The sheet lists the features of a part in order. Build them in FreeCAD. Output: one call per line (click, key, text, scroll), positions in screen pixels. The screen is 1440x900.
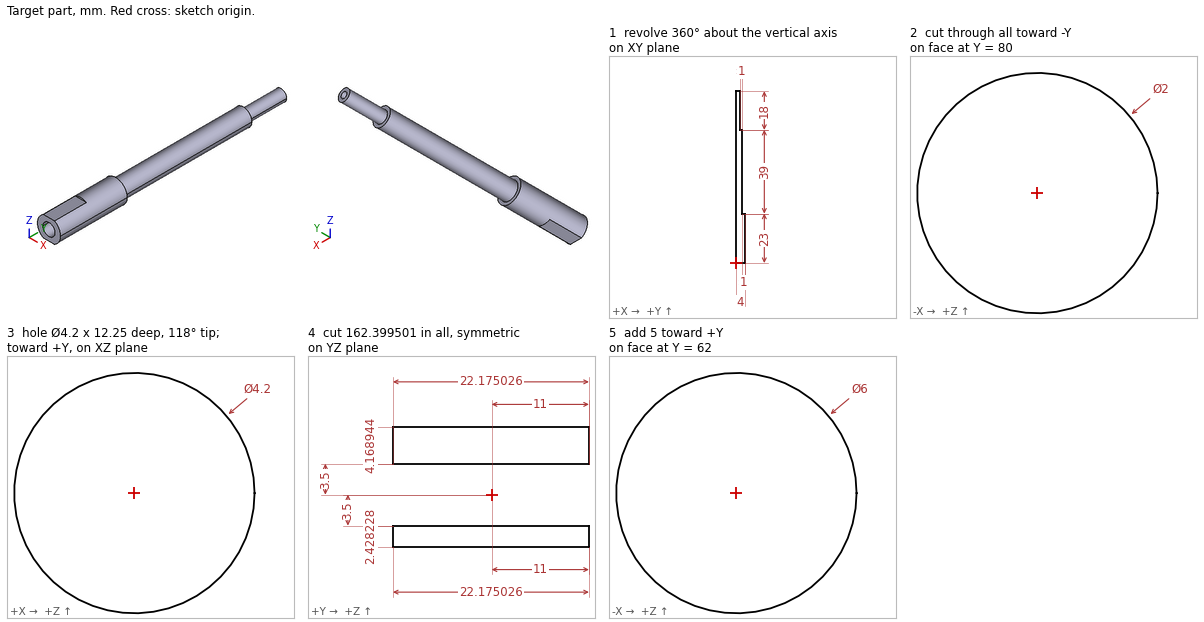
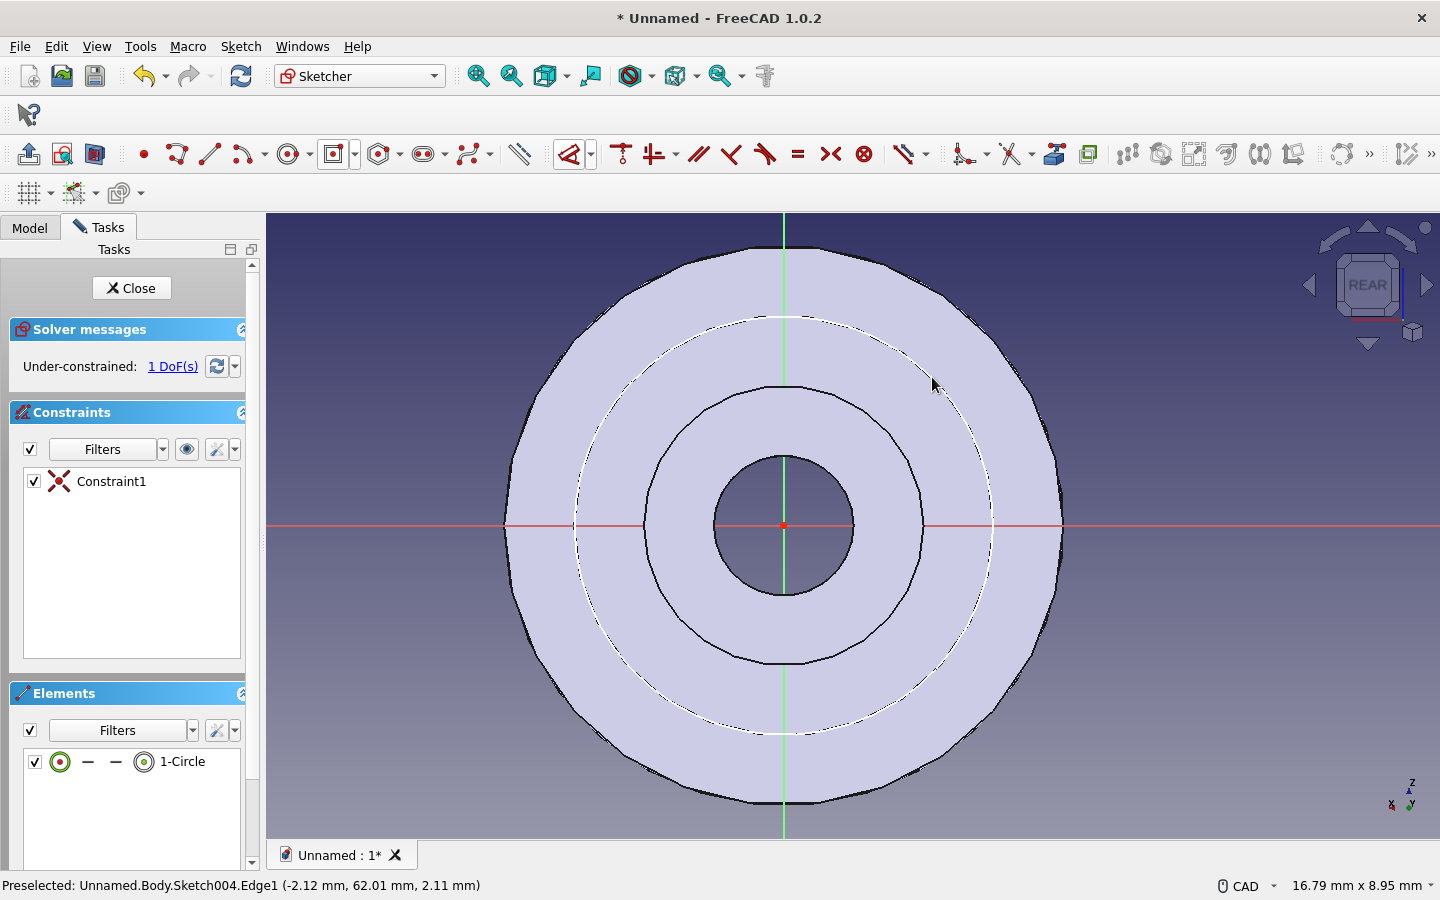
click(931, 377)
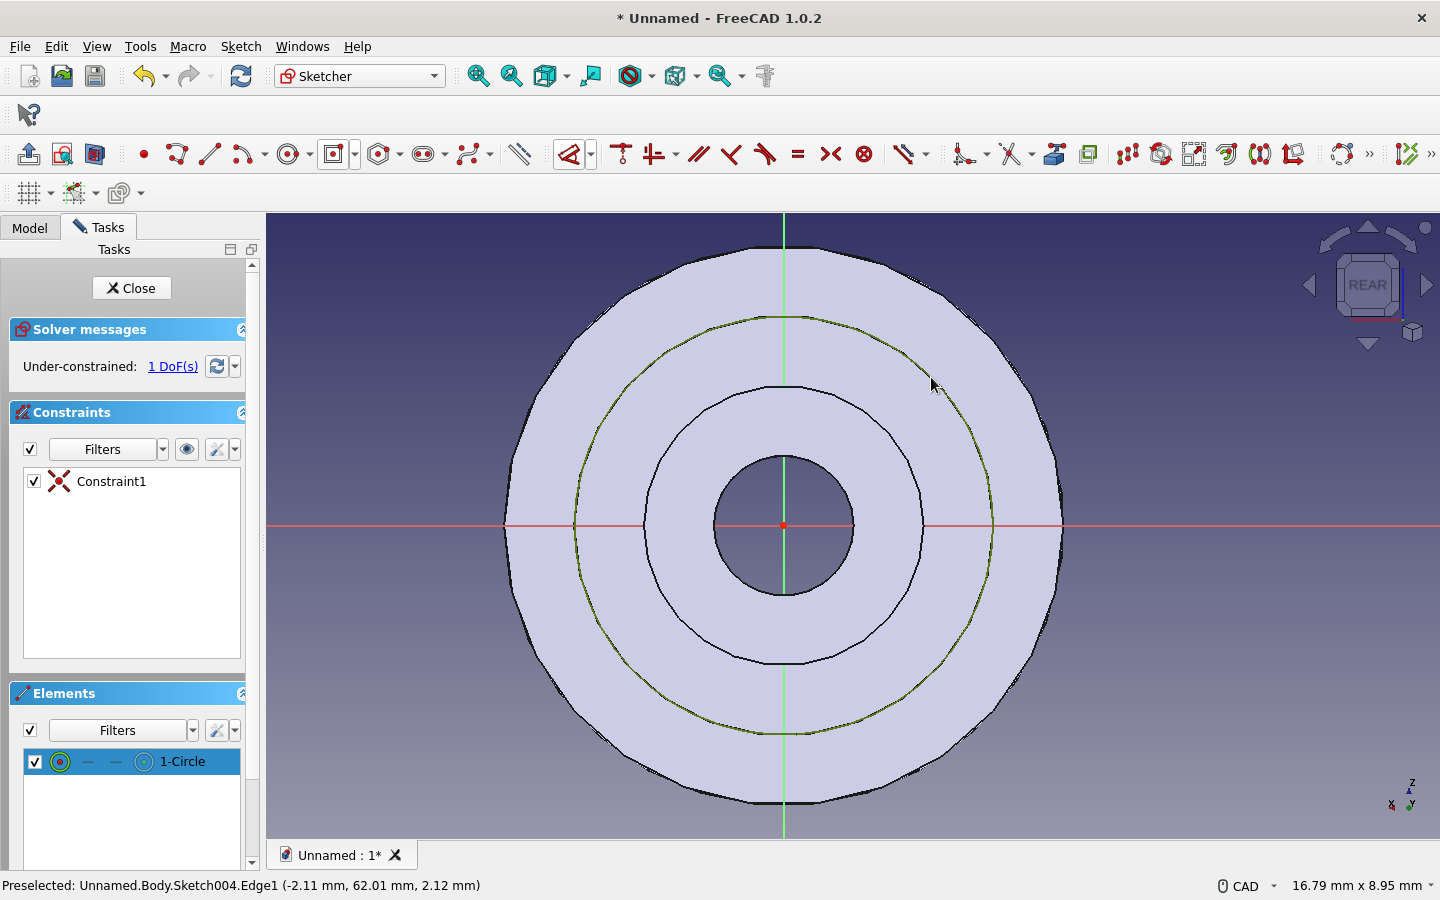
key(k)
key(o)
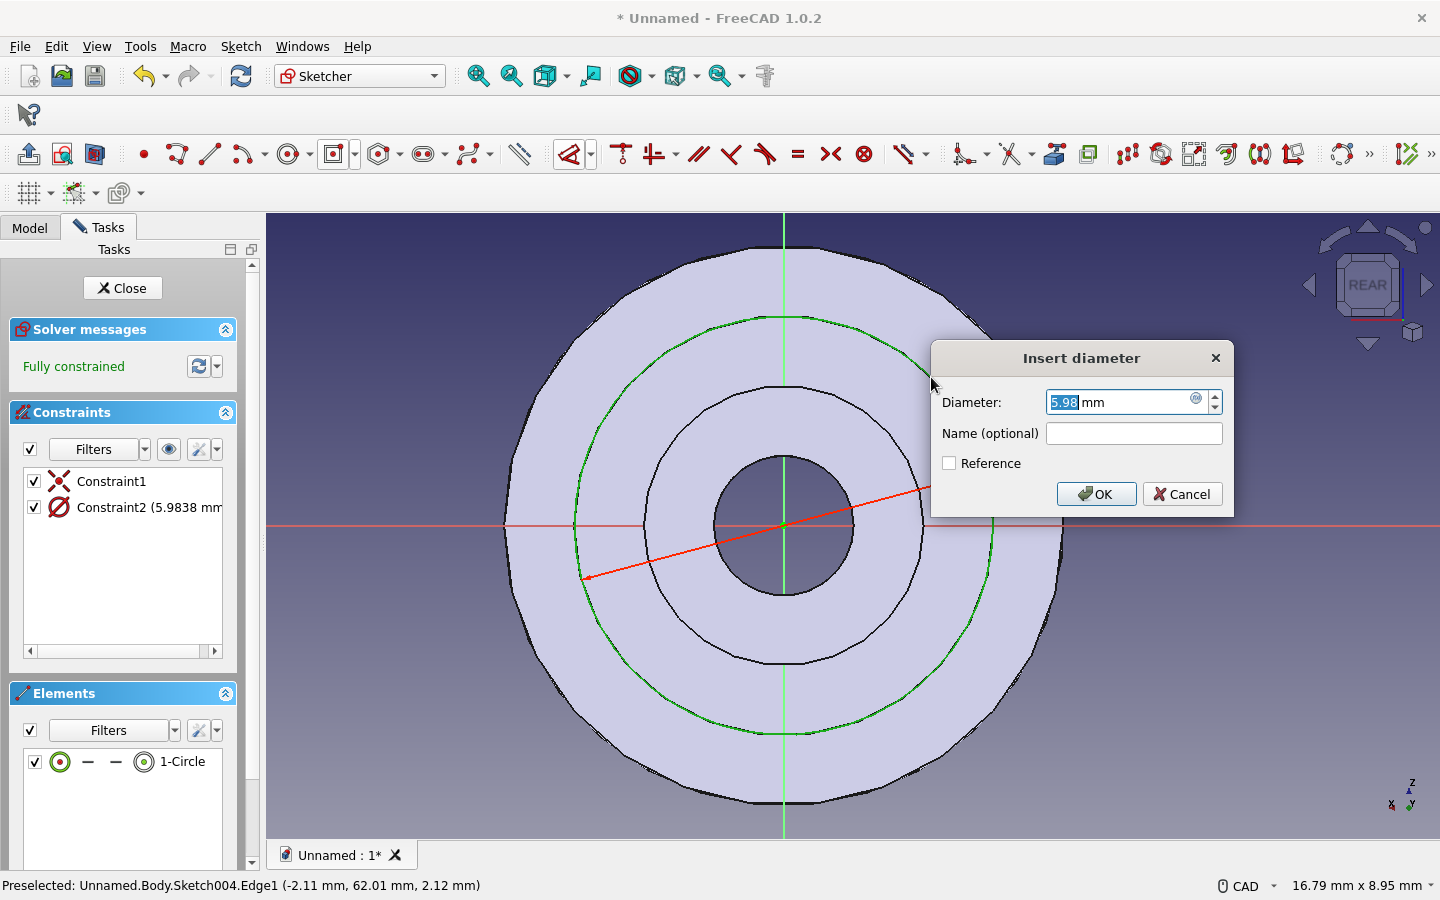
text(6)
key(Return)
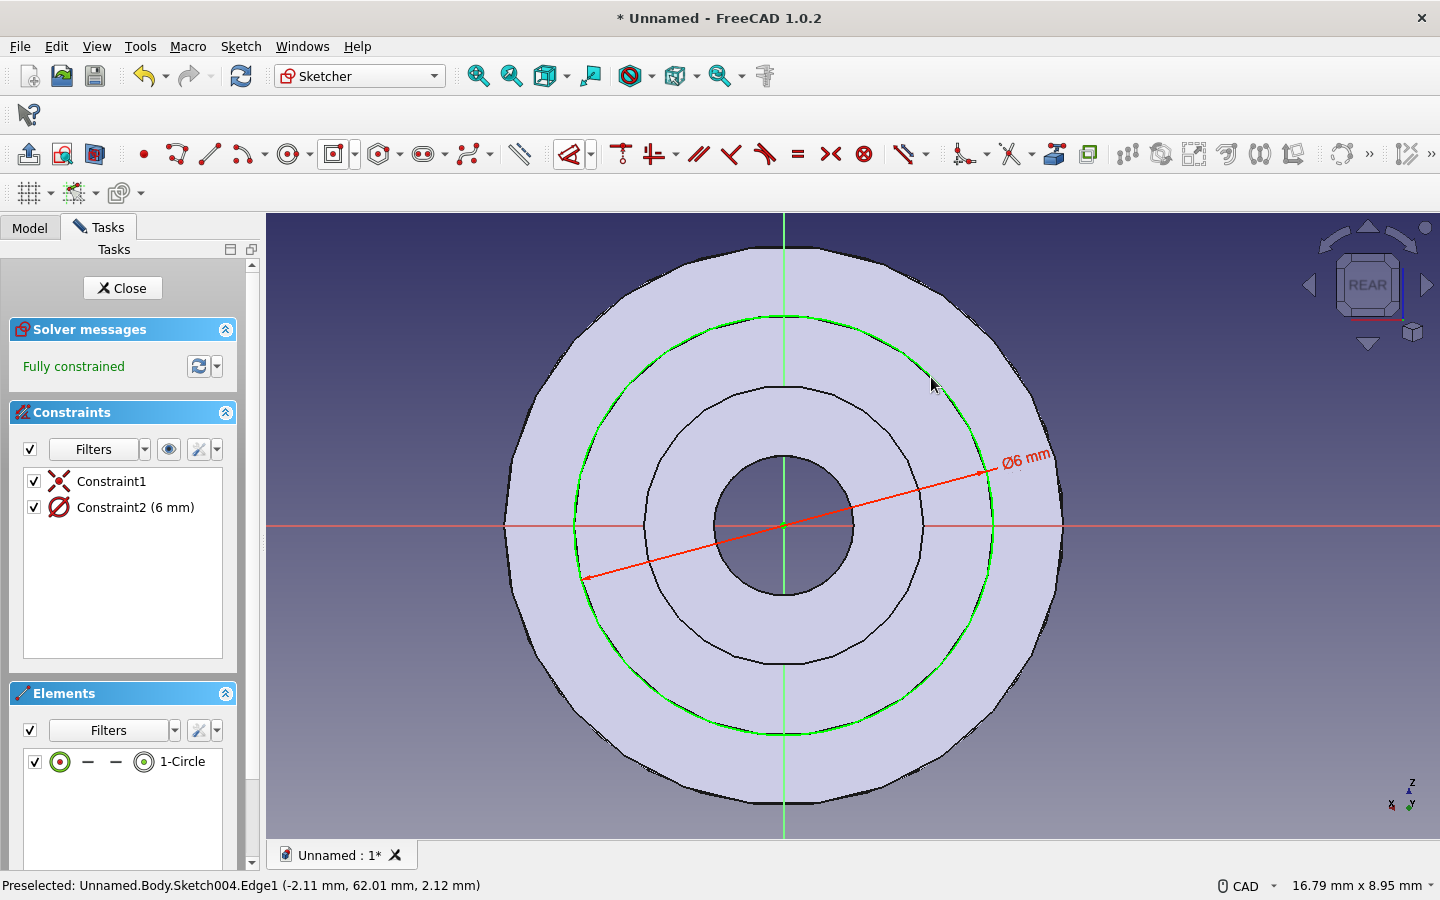
click(123, 288)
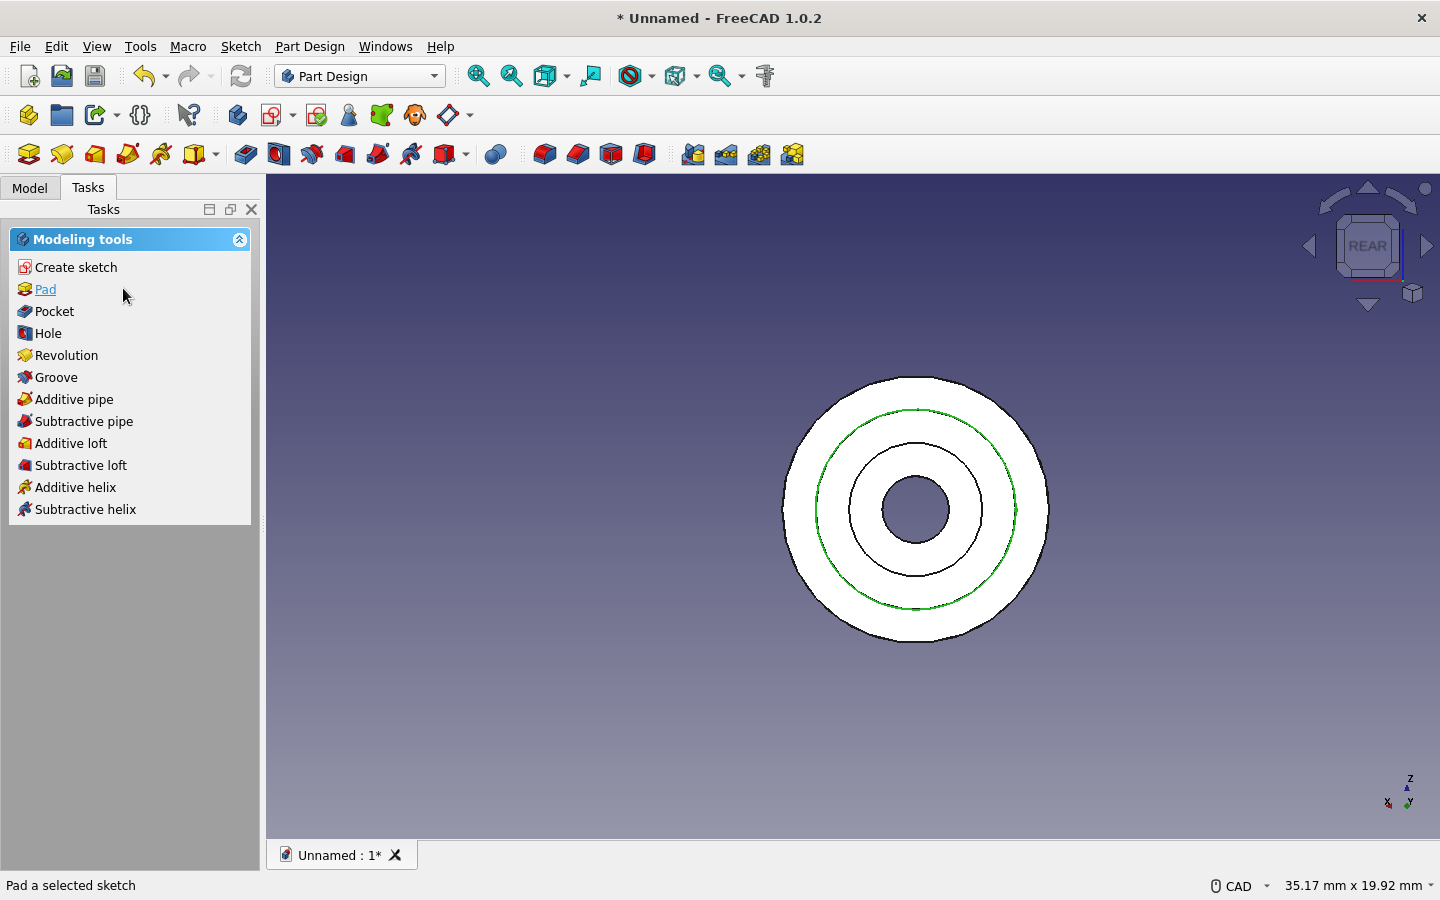
click(29, 154)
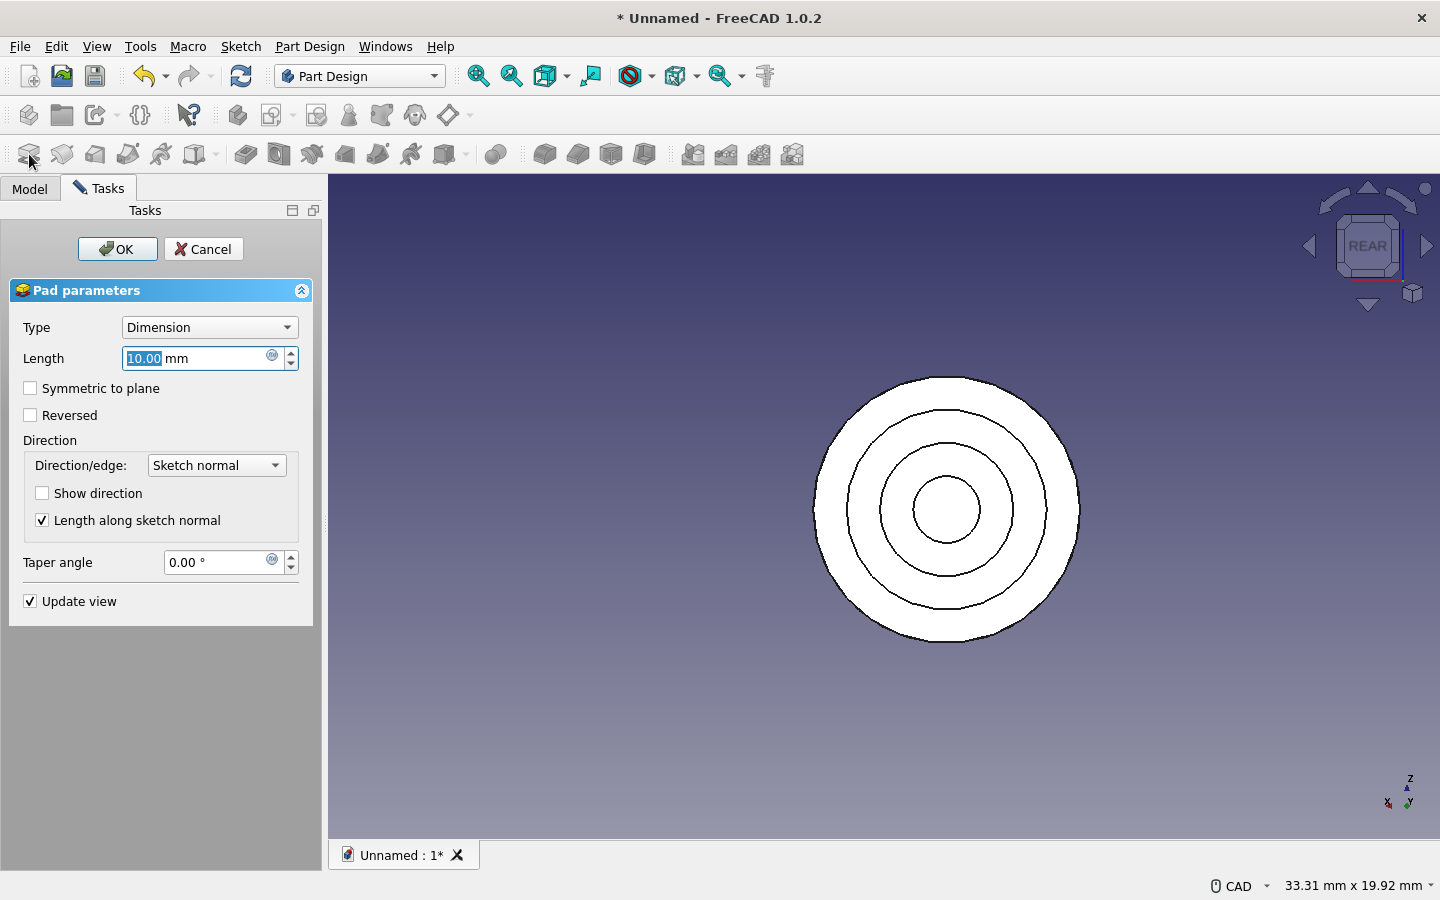
text(5)
key(Tab)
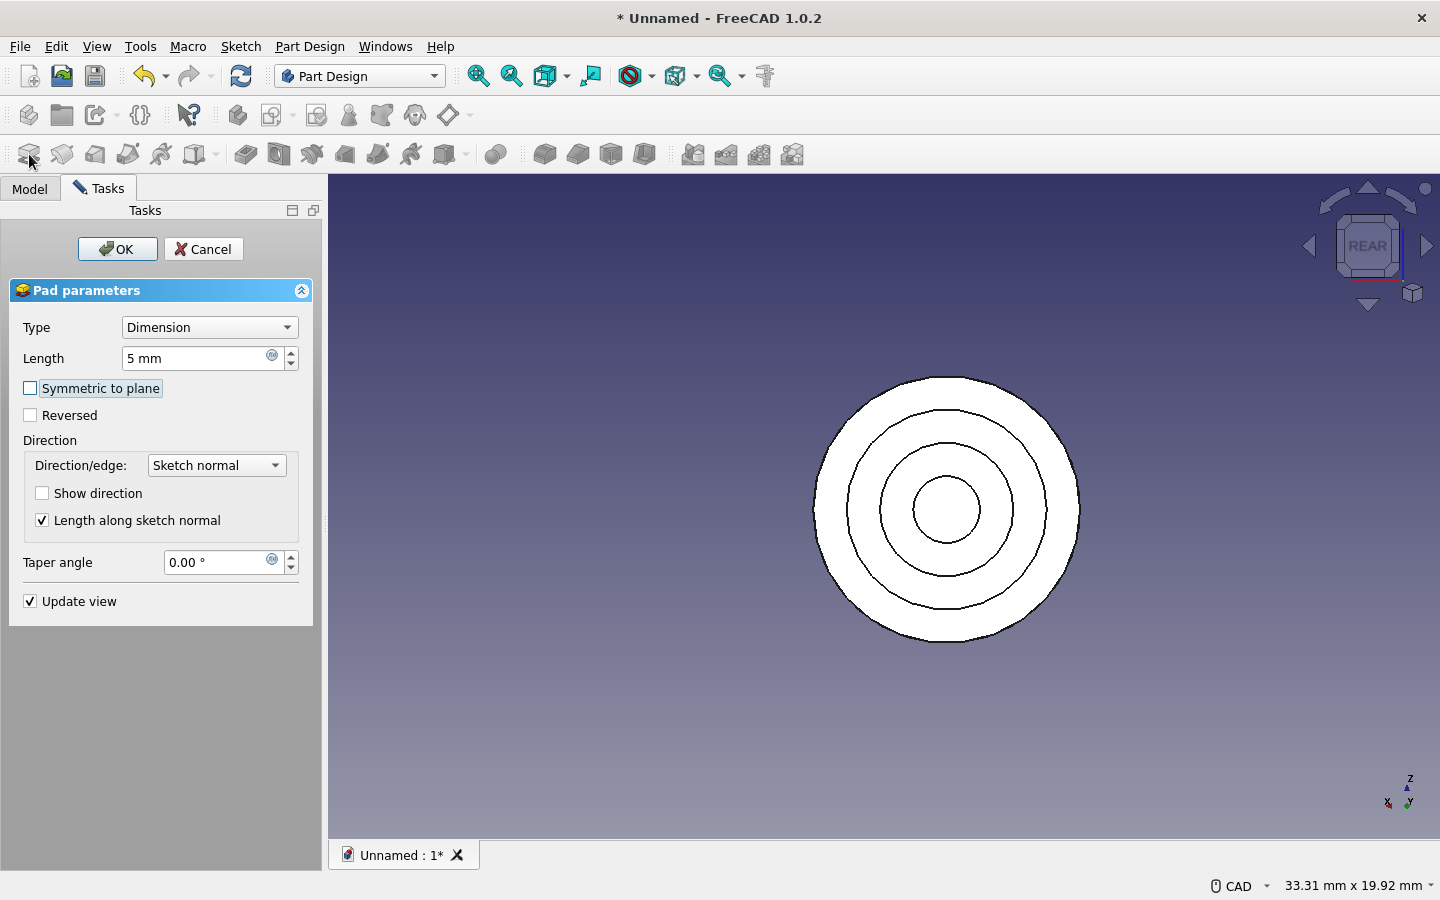
click(118, 249)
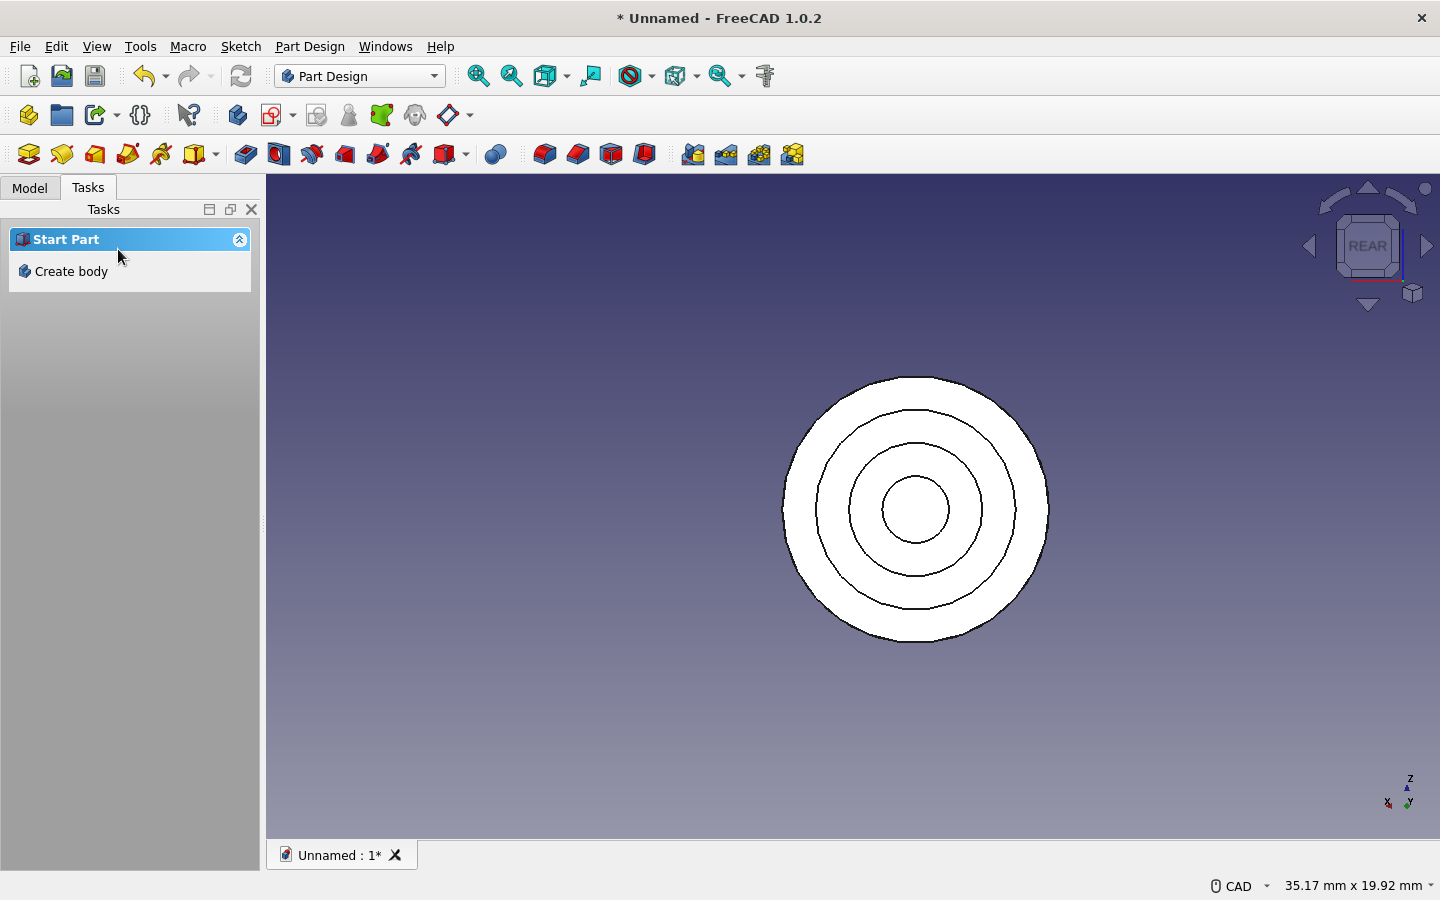
key(0)